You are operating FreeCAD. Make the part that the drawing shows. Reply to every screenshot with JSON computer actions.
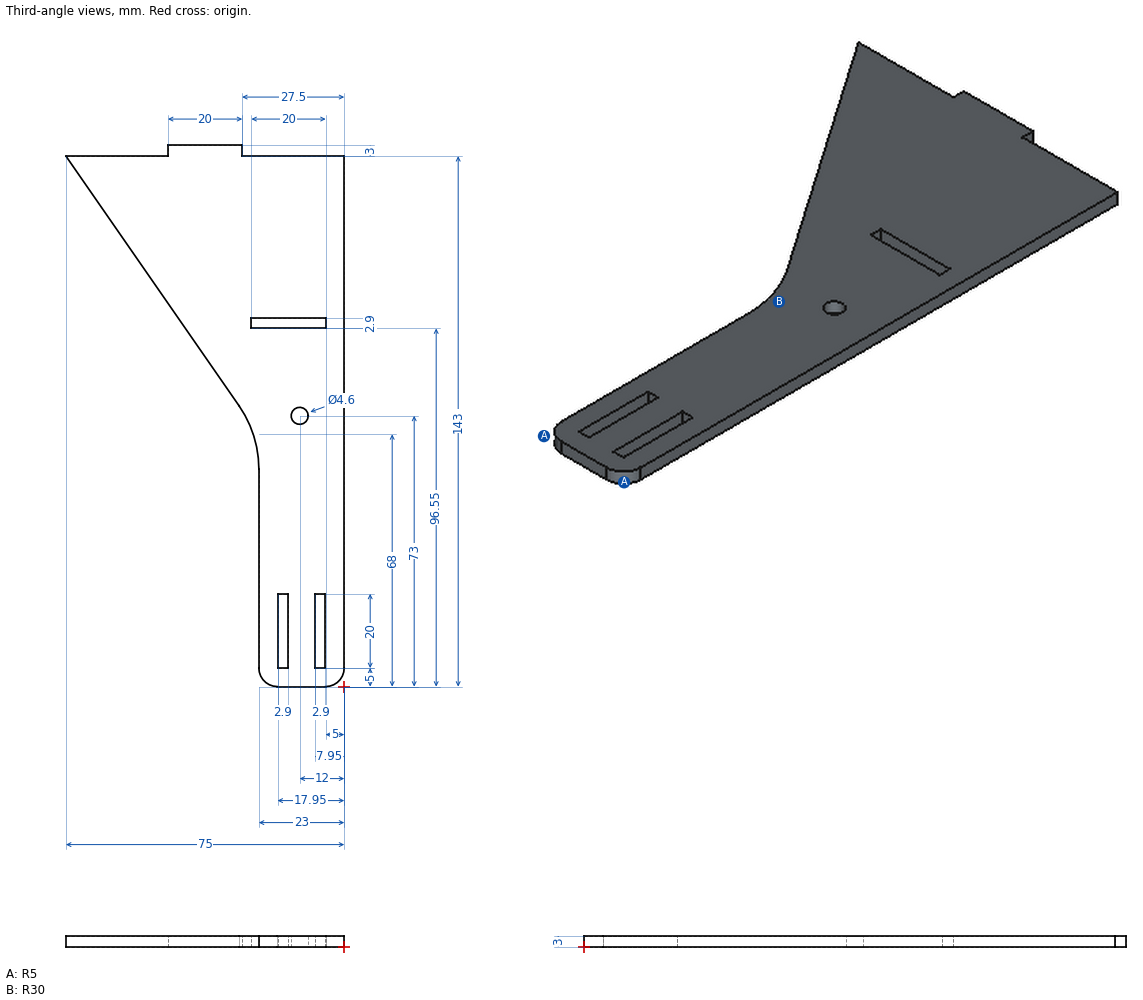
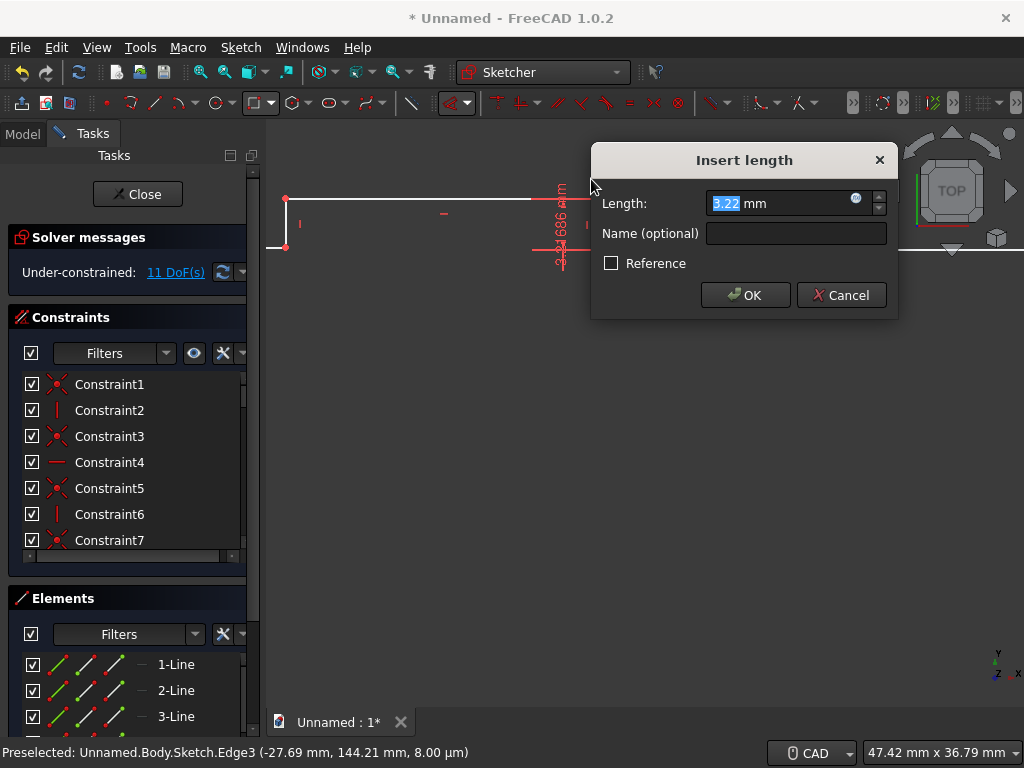
{"action": "type", "text": "3"}
{"action": "key", "text": "Return"}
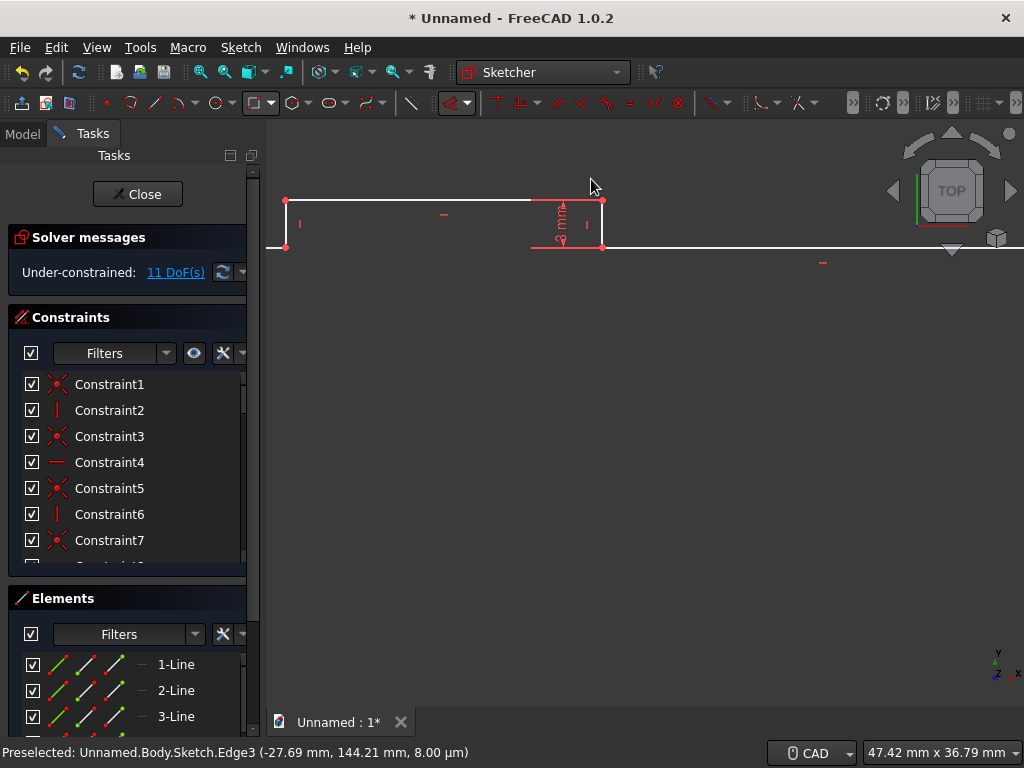
{"action": "scroll", "coordinate": [602, 225], "scroll_direction": "down", "scroll_amount": 9}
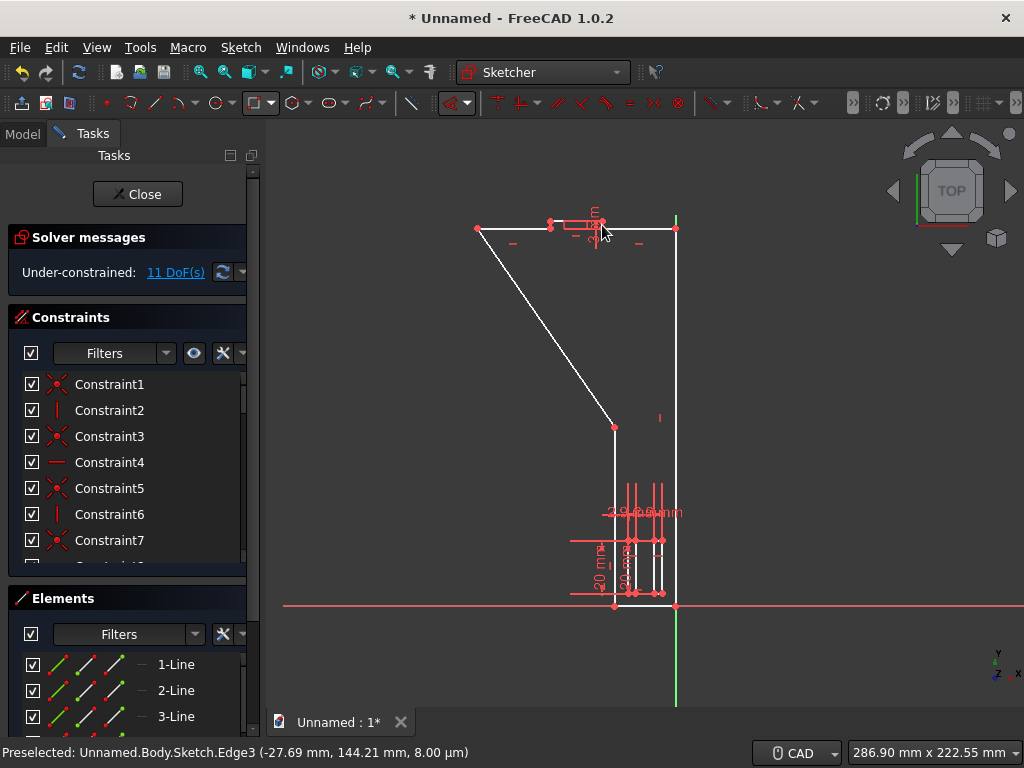
{"action": "scroll", "coordinate": [550, 223], "scroll_direction": "up", "scroll_amount": 9}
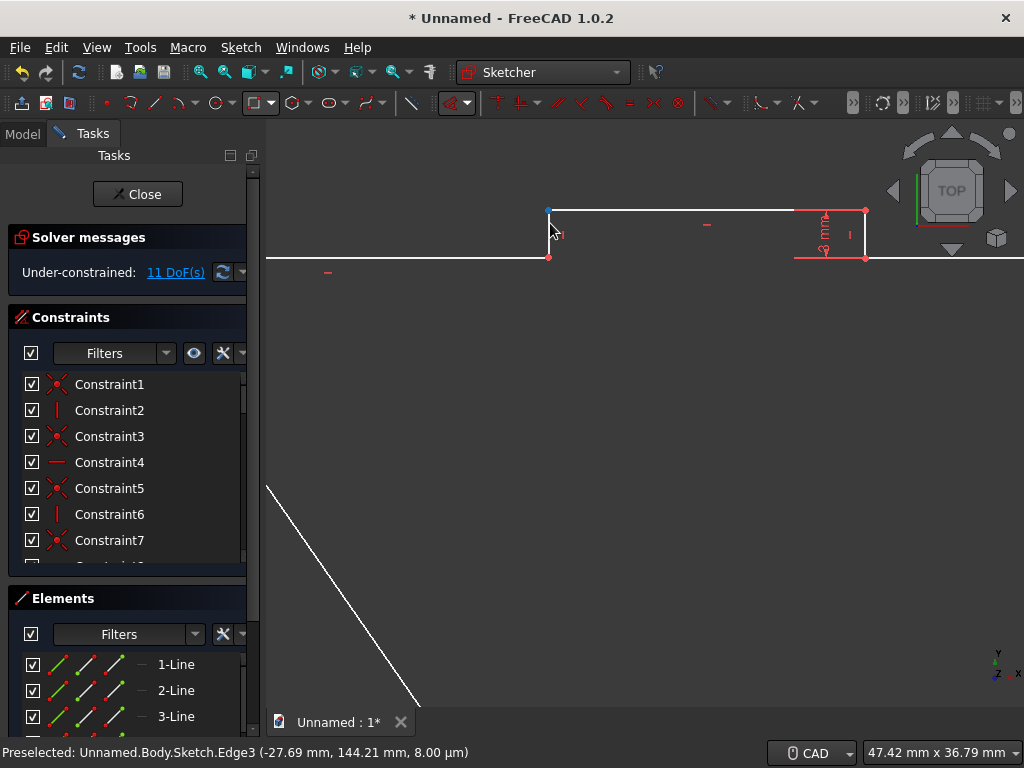
{"action": "left_click", "coordinate": [549, 224]}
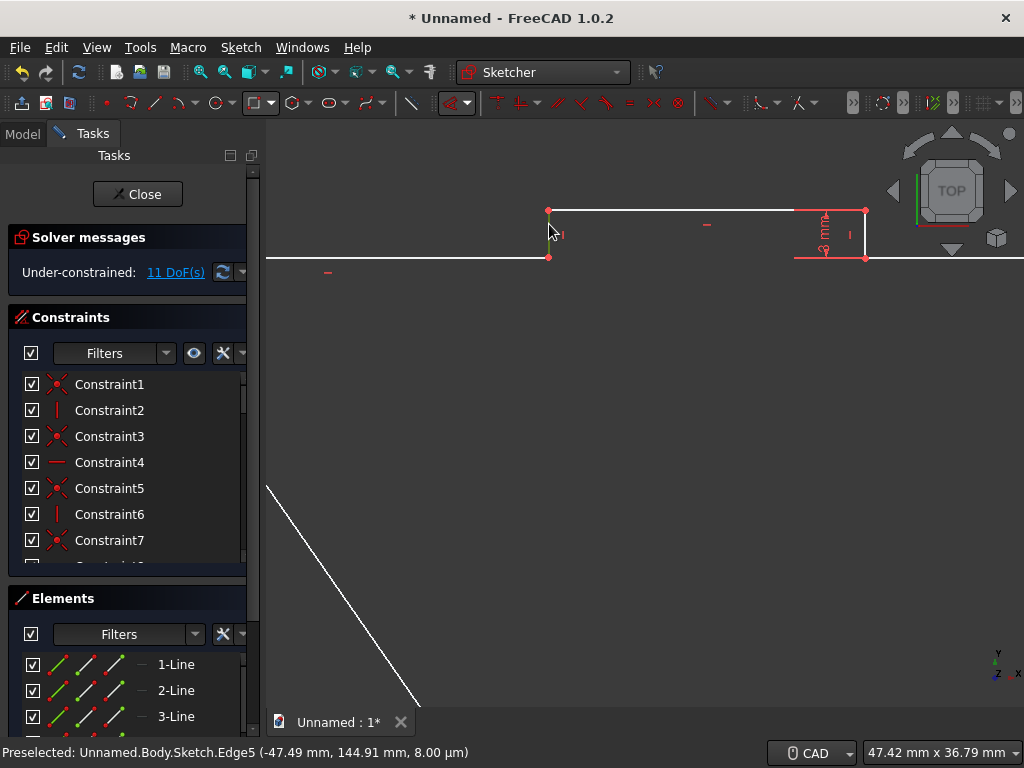
{"action": "key", "text": "i"}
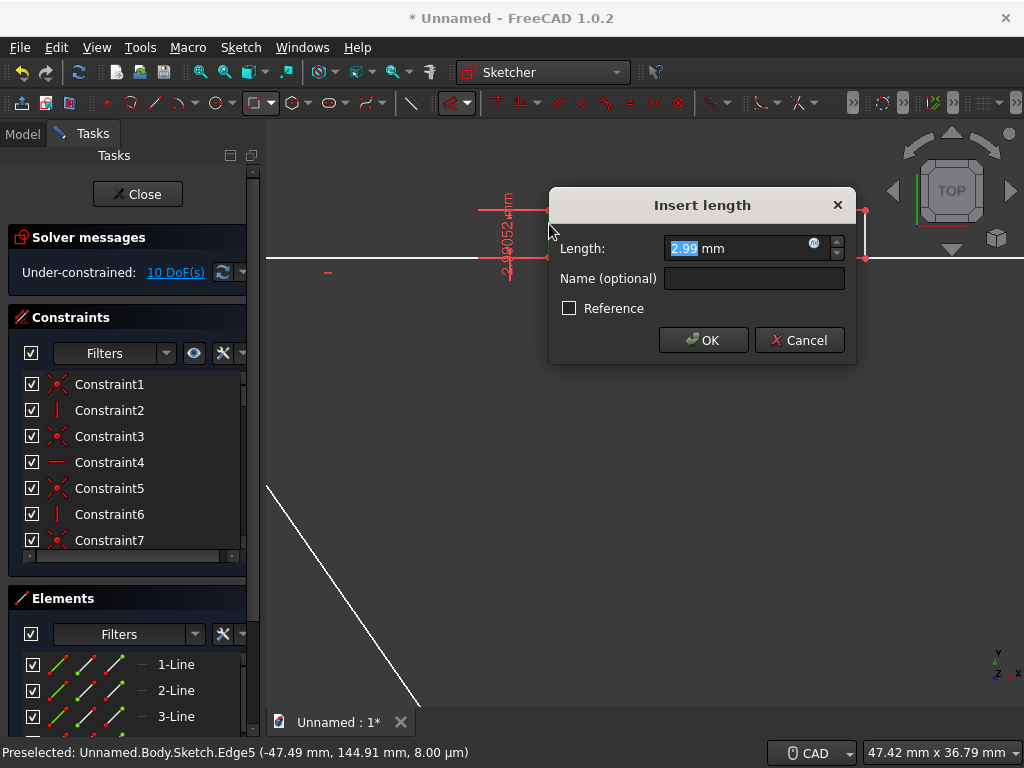
{"action": "type", "text": "3"}
{"action": "key", "text": "Return"}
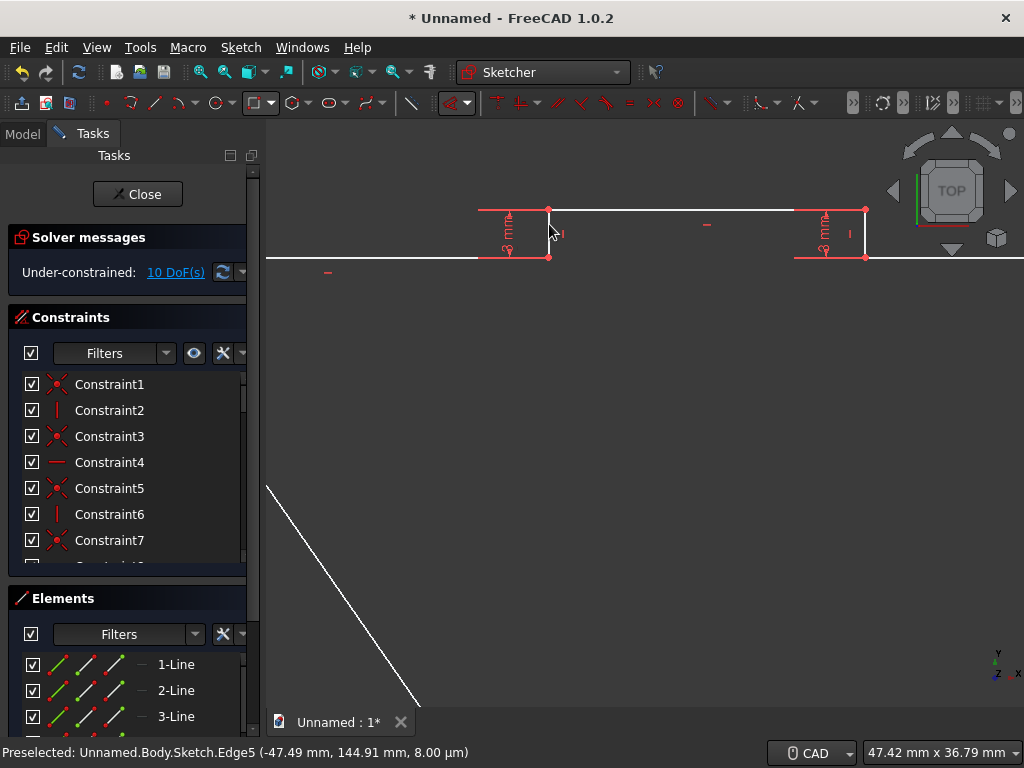
{"action": "scroll", "coordinate": [550, 223], "scroll_direction": "down", "scroll_amount": 9}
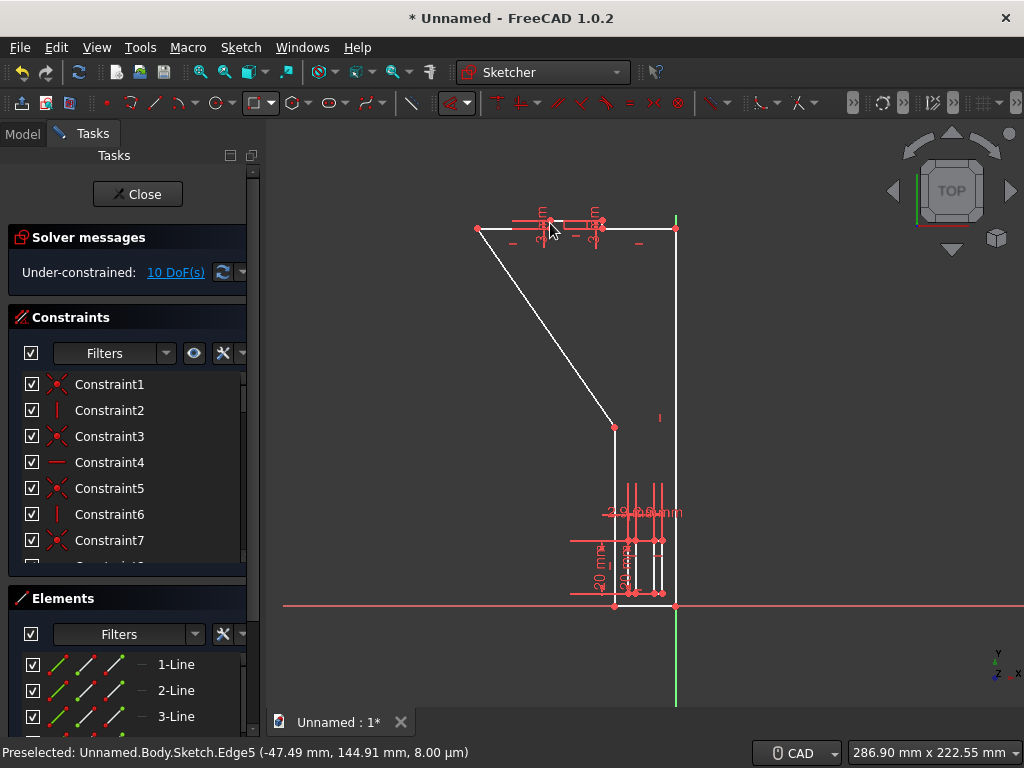
{"action": "left_click", "coordinate": [571, 221]}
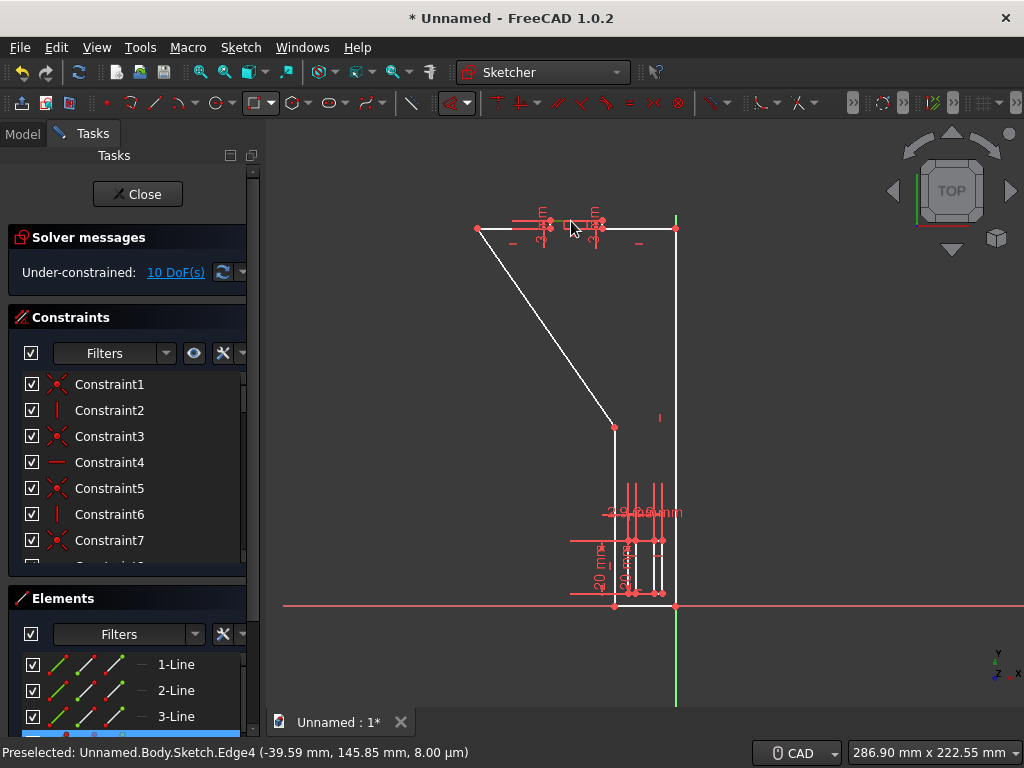
{"action": "left_click", "coordinate": [470, 104]}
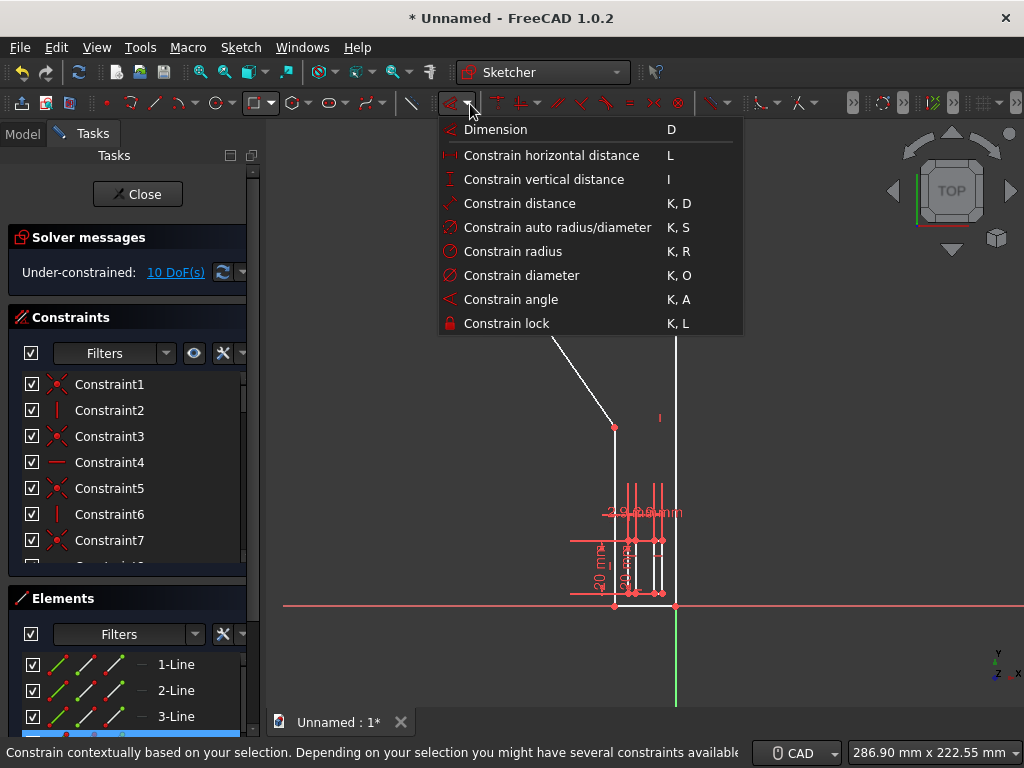
{"action": "left_click", "coordinate": [591, 155]}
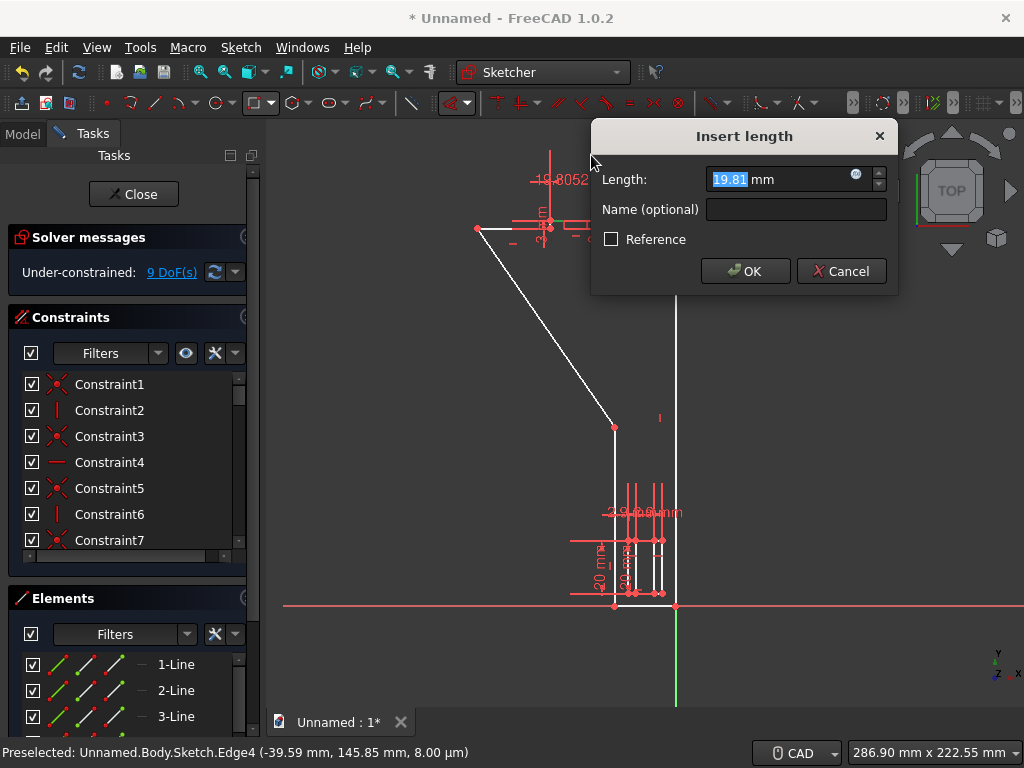
{"action": "type", "text": "20"}
{"action": "key", "text": "Return"}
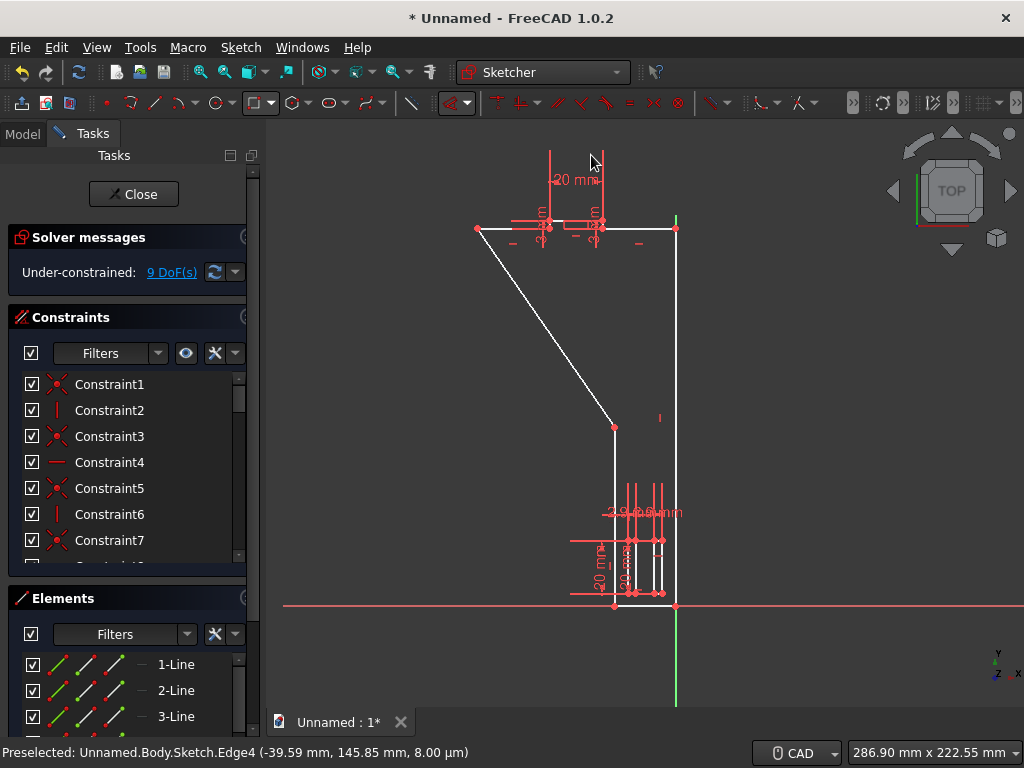
{"action": "left_click", "coordinate": [615, 481]}